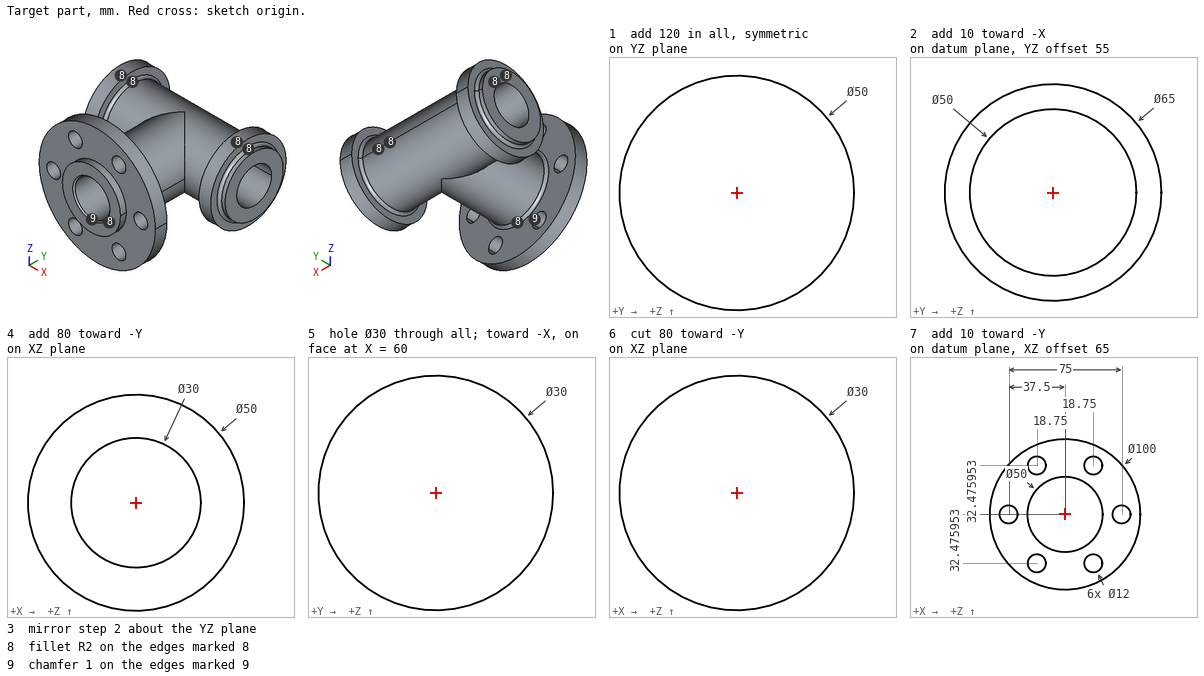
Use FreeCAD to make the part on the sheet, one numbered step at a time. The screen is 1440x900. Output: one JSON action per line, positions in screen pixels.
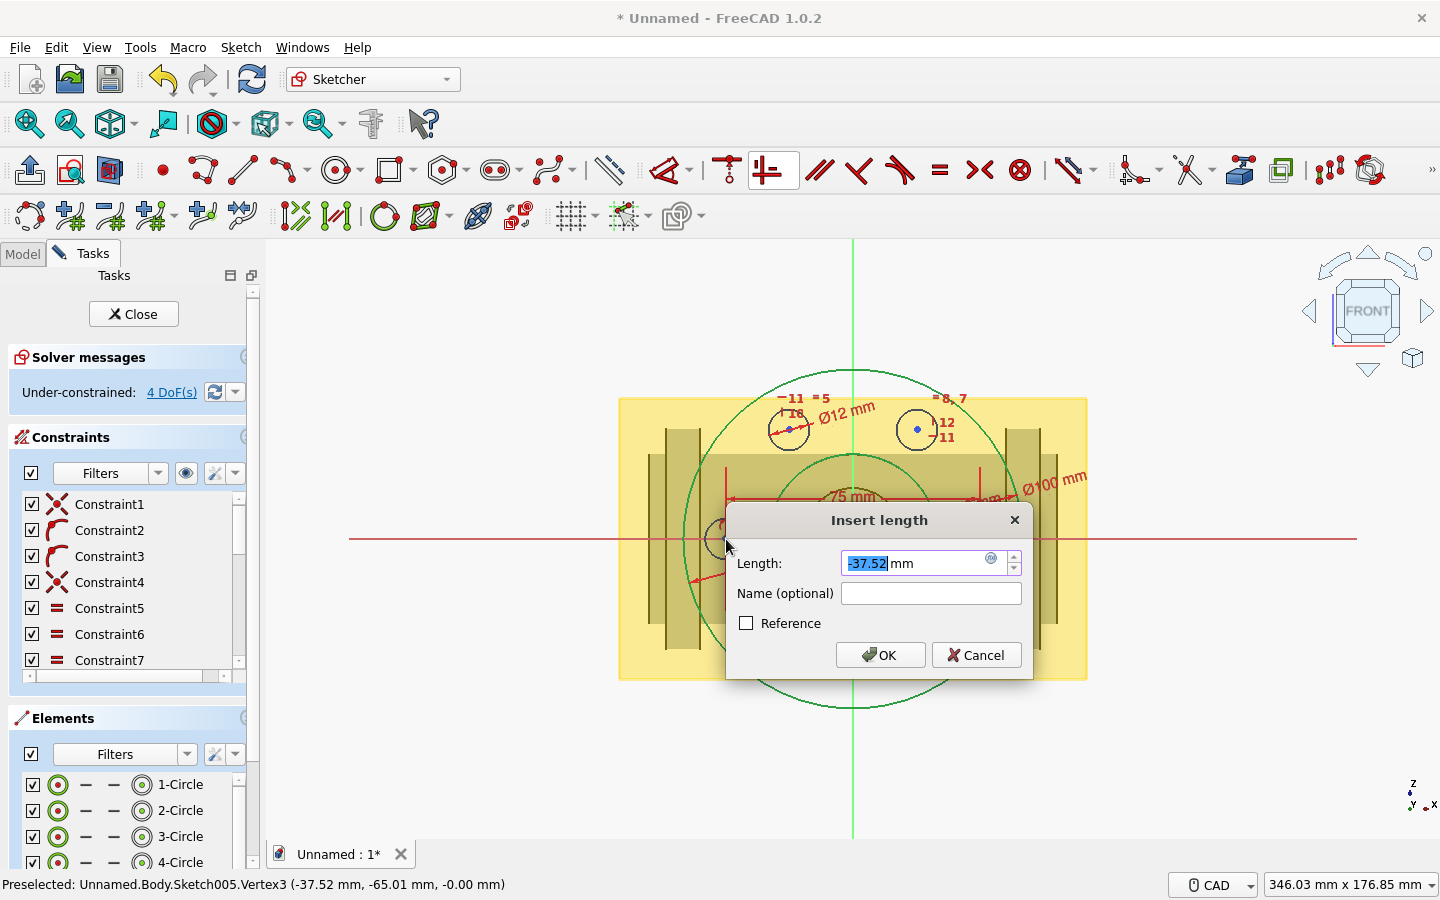
{"action": "type", "text": "-37.5"}
{"action": "key", "text": "Return"}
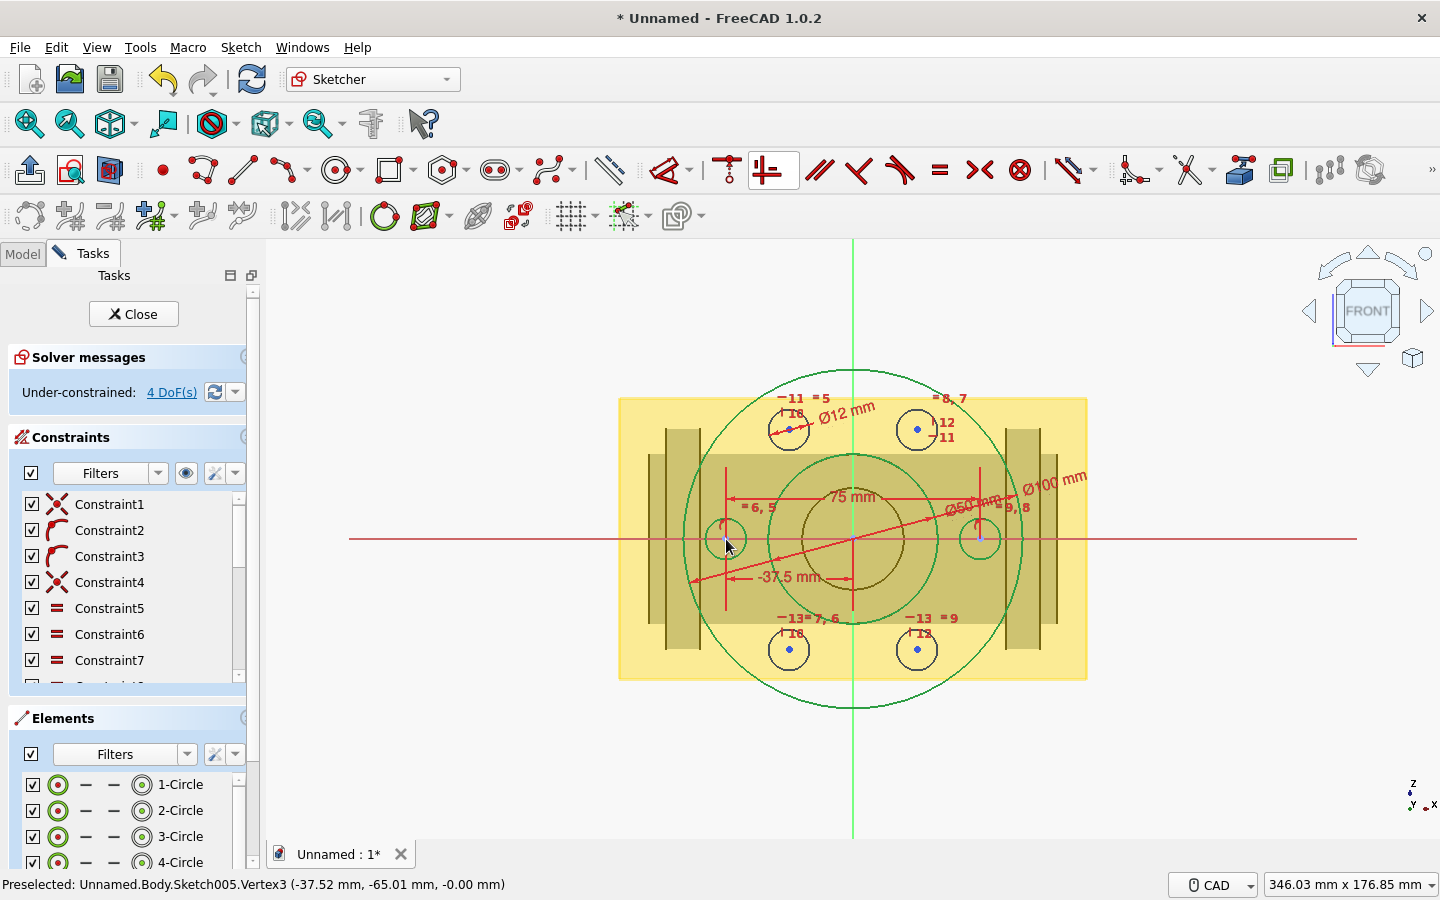
{"action": "left_click", "coordinate": [789, 430]}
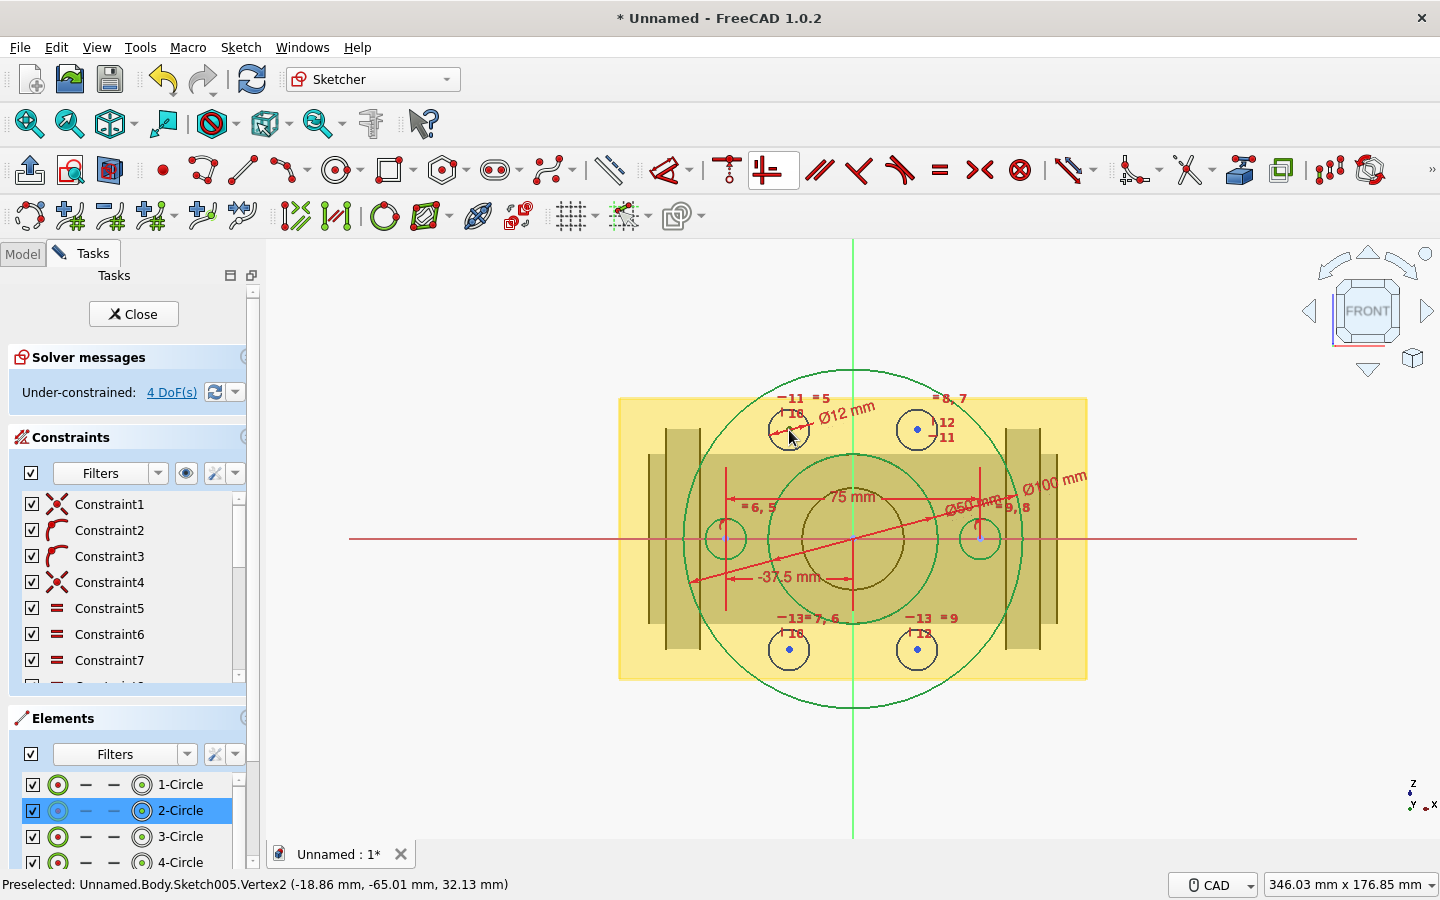
{"action": "key", "text": "l"}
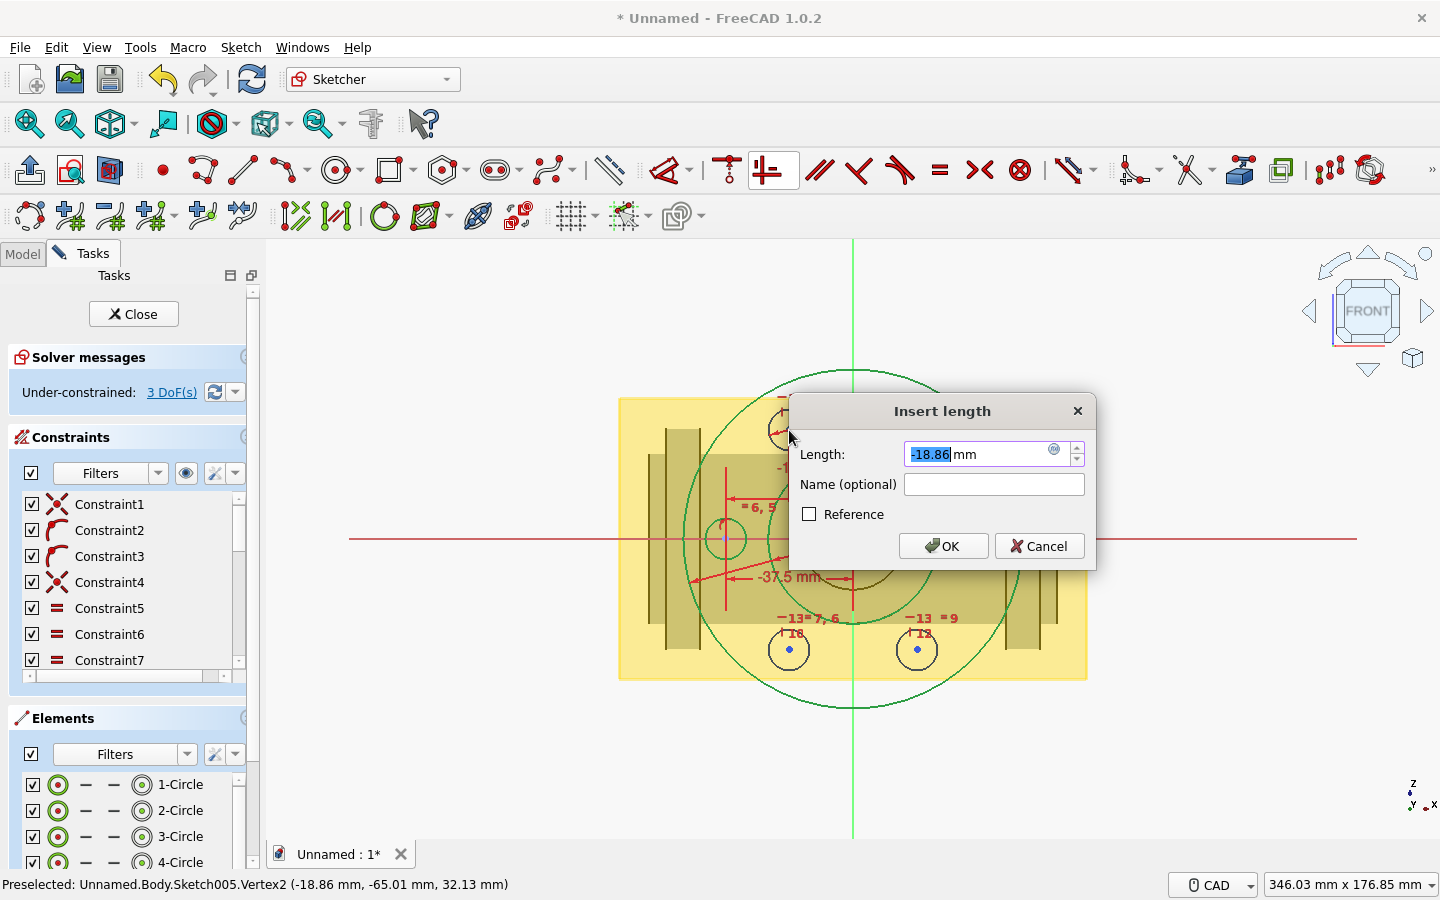
{"action": "type", "text": "-18.75"}
{"action": "key", "text": "Return"}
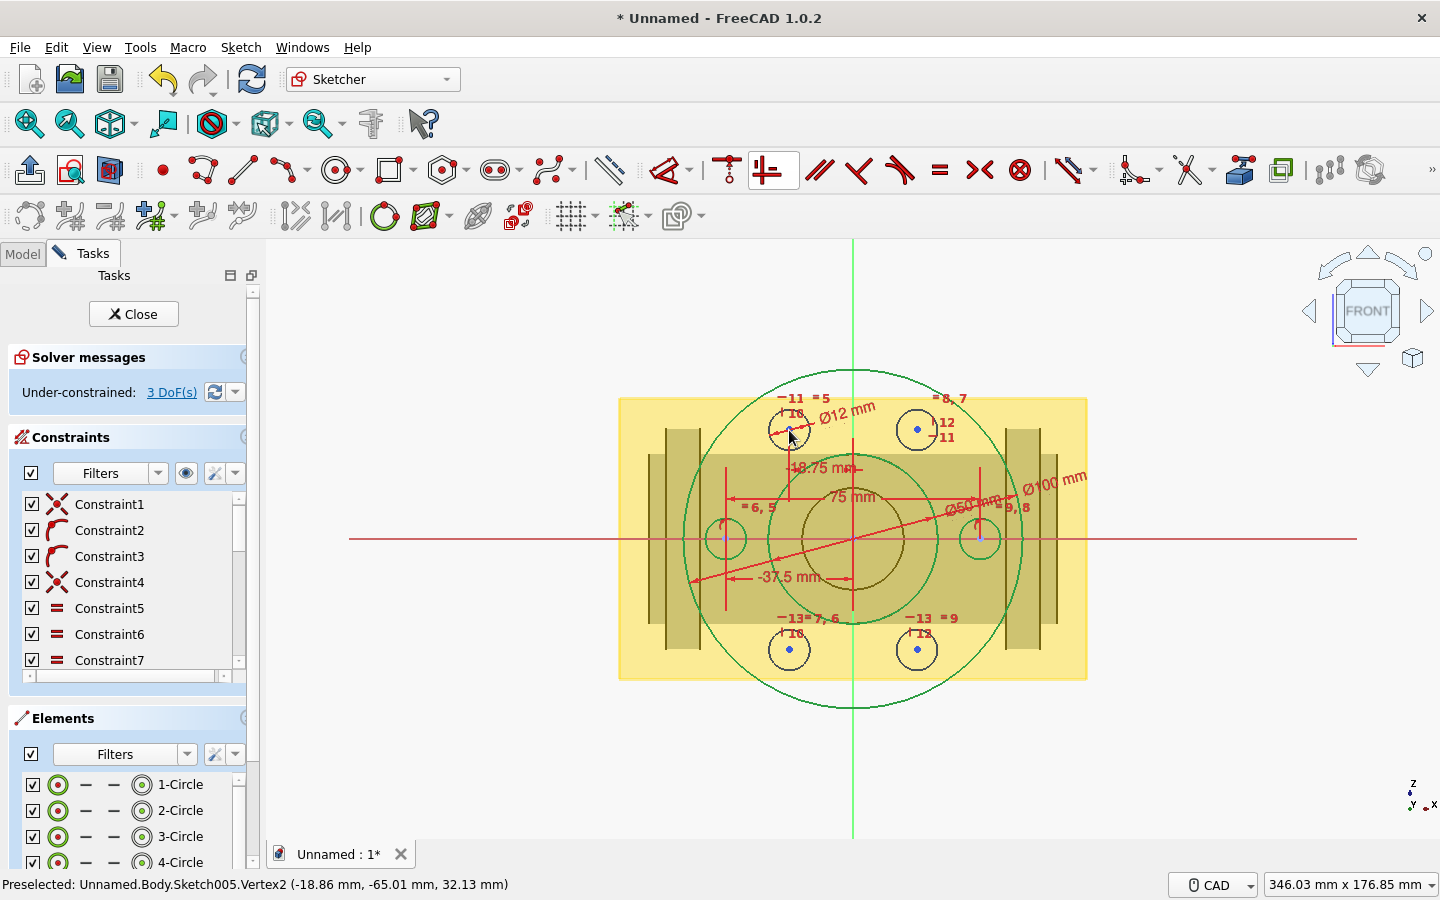
{"action": "left_click", "coordinate": [917, 430]}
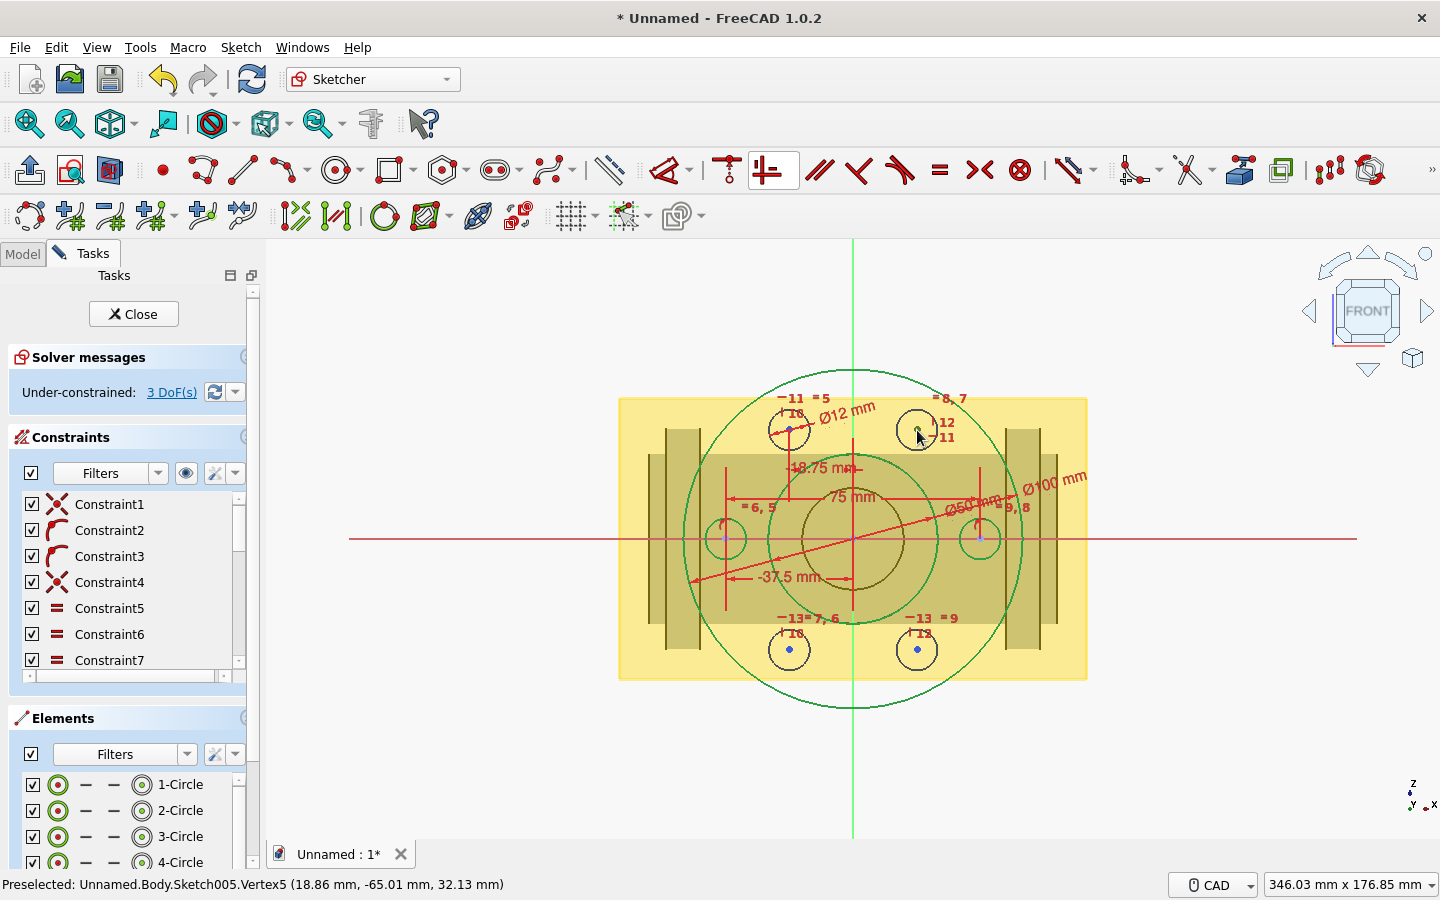
{"action": "left_click", "coordinate": [692, 170]}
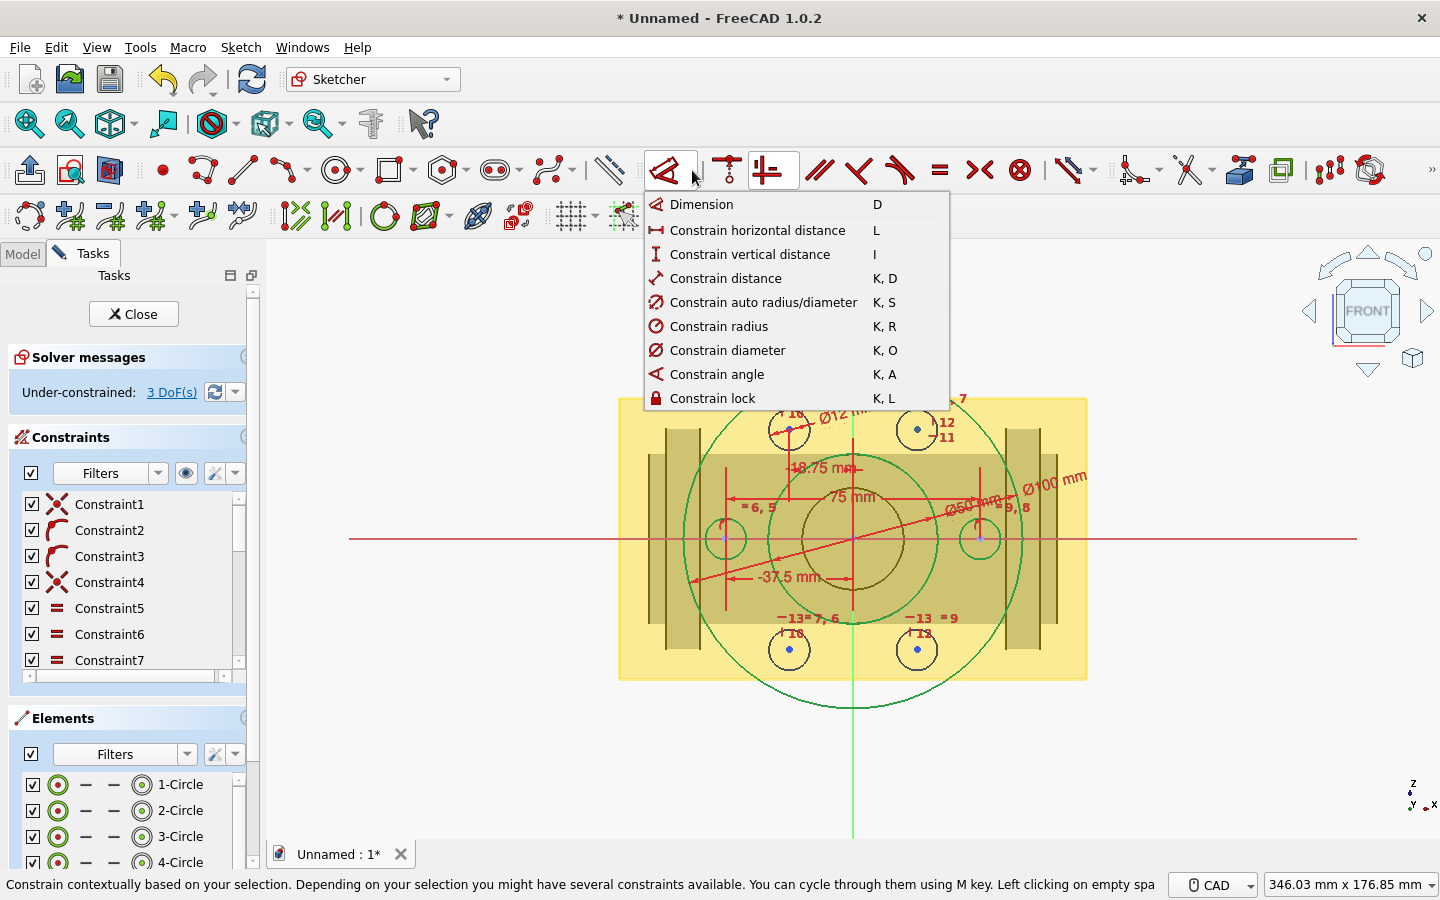
{"action": "left_click", "coordinate": [797, 230]}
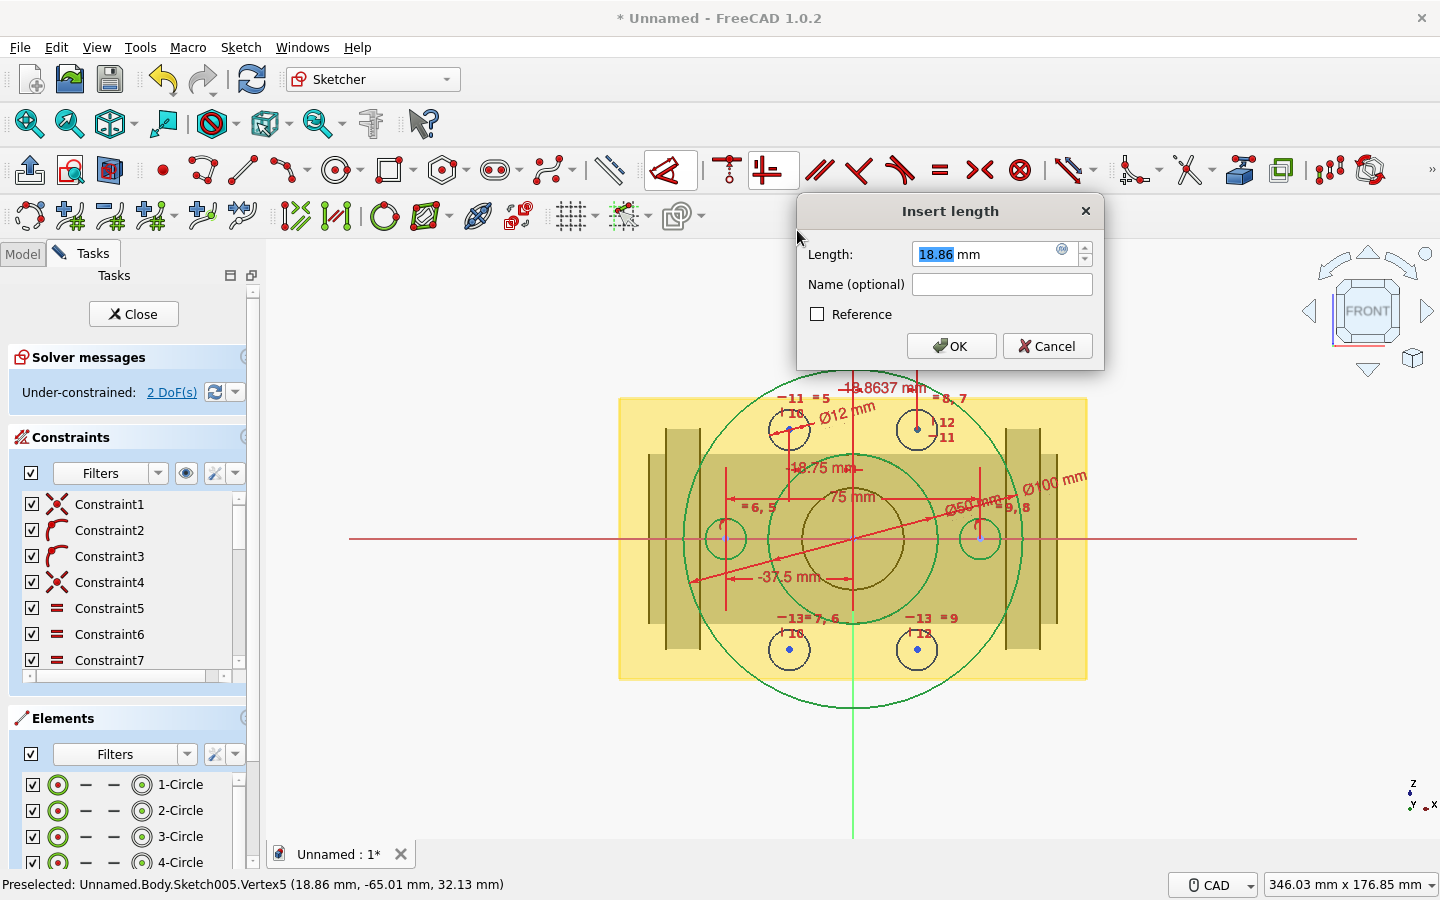
{"action": "type", "text": "18.75"}
{"action": "key", "text": "Return"}